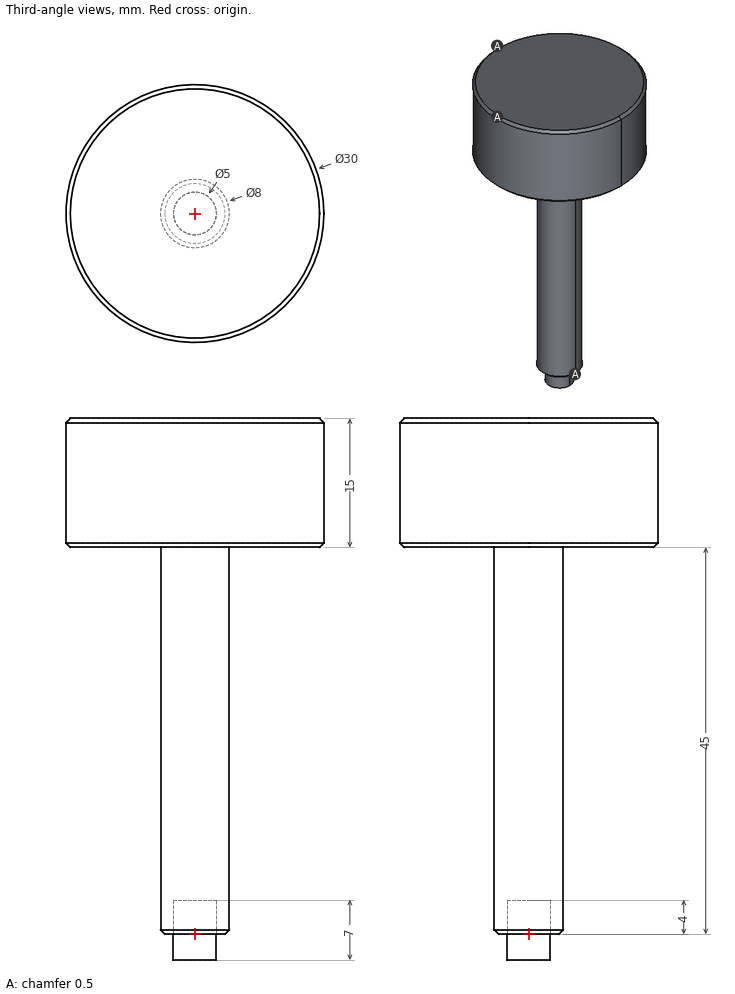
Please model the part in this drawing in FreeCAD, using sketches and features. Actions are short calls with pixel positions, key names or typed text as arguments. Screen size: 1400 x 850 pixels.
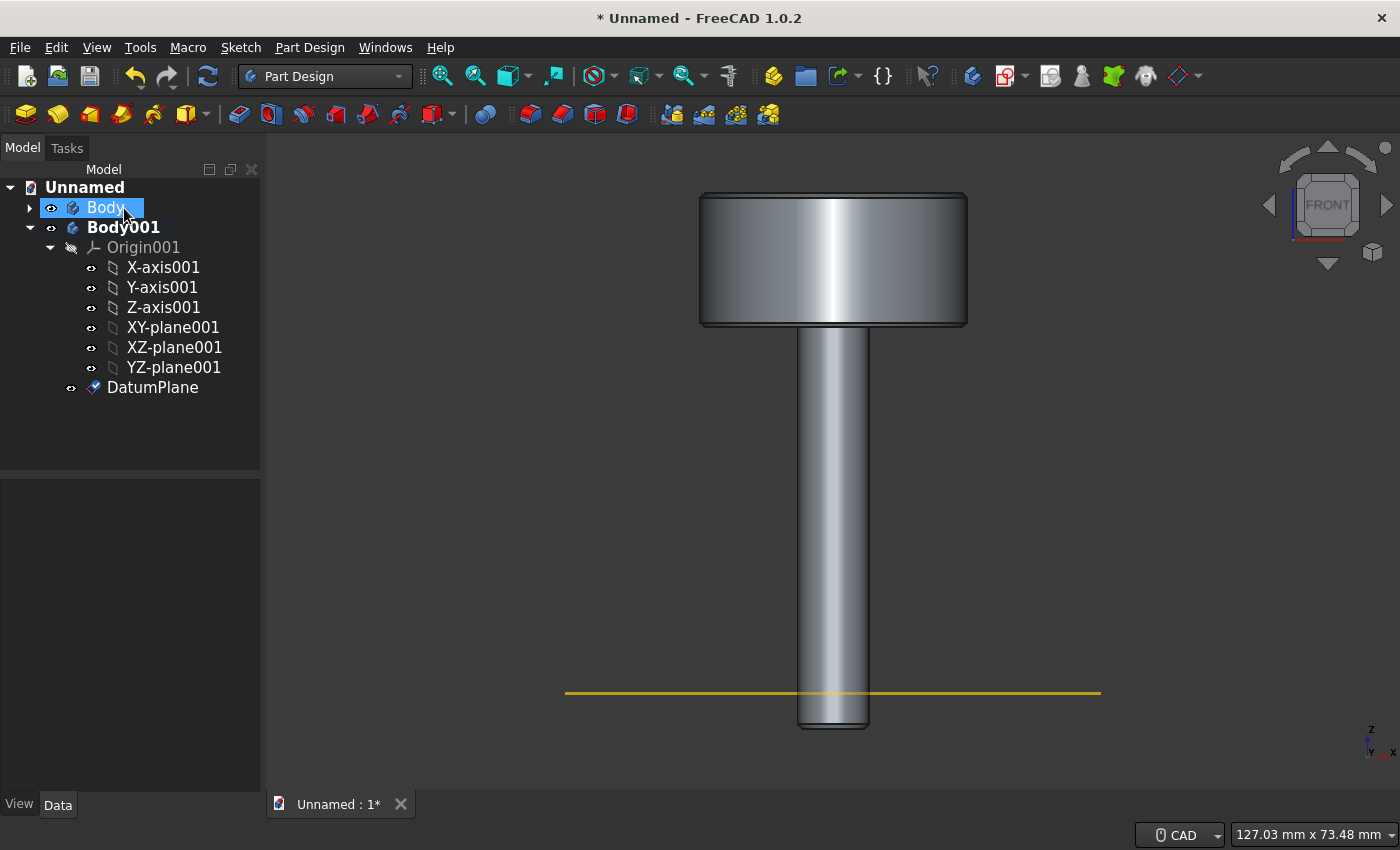
click(116, 388)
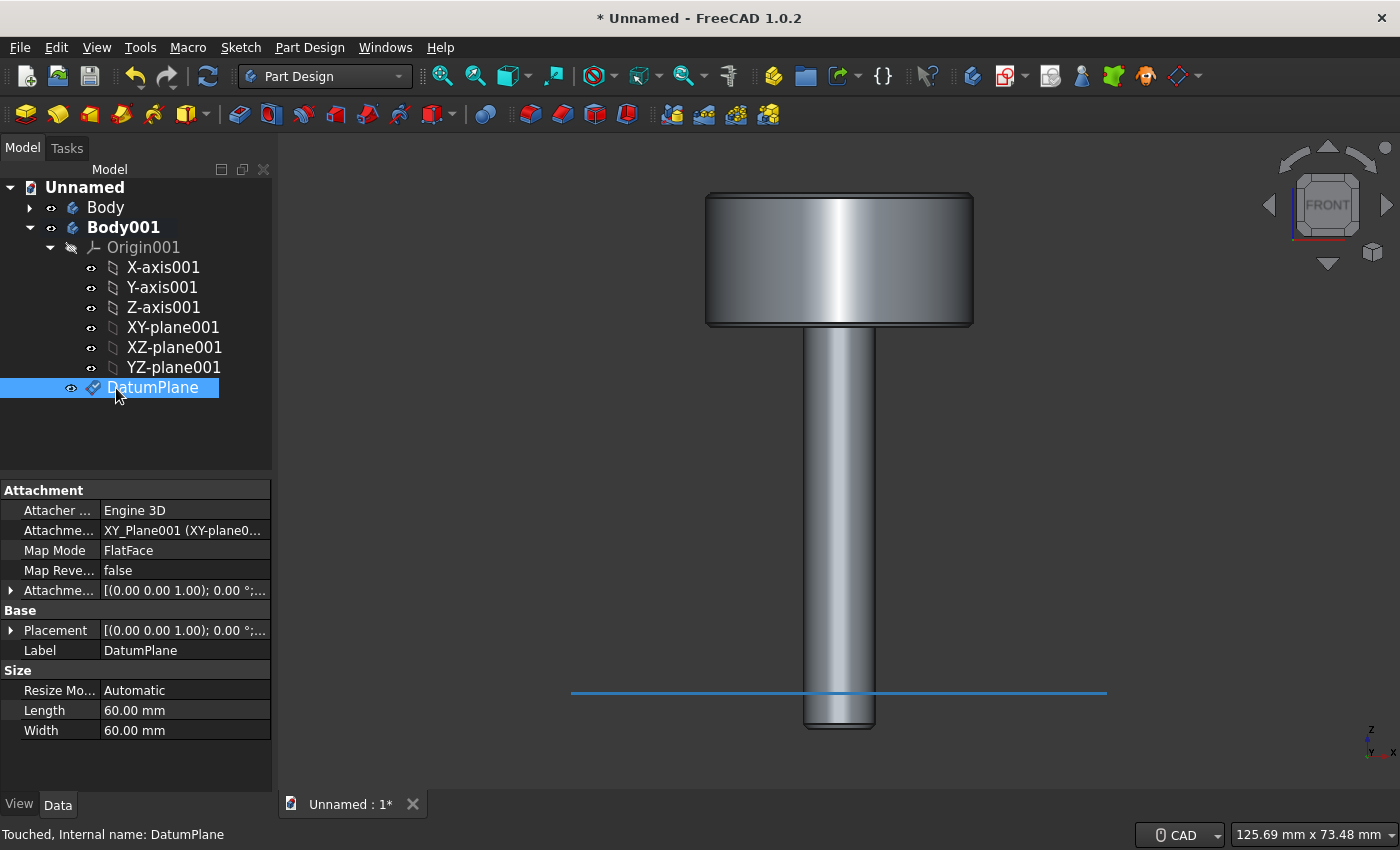
click(1006, 76)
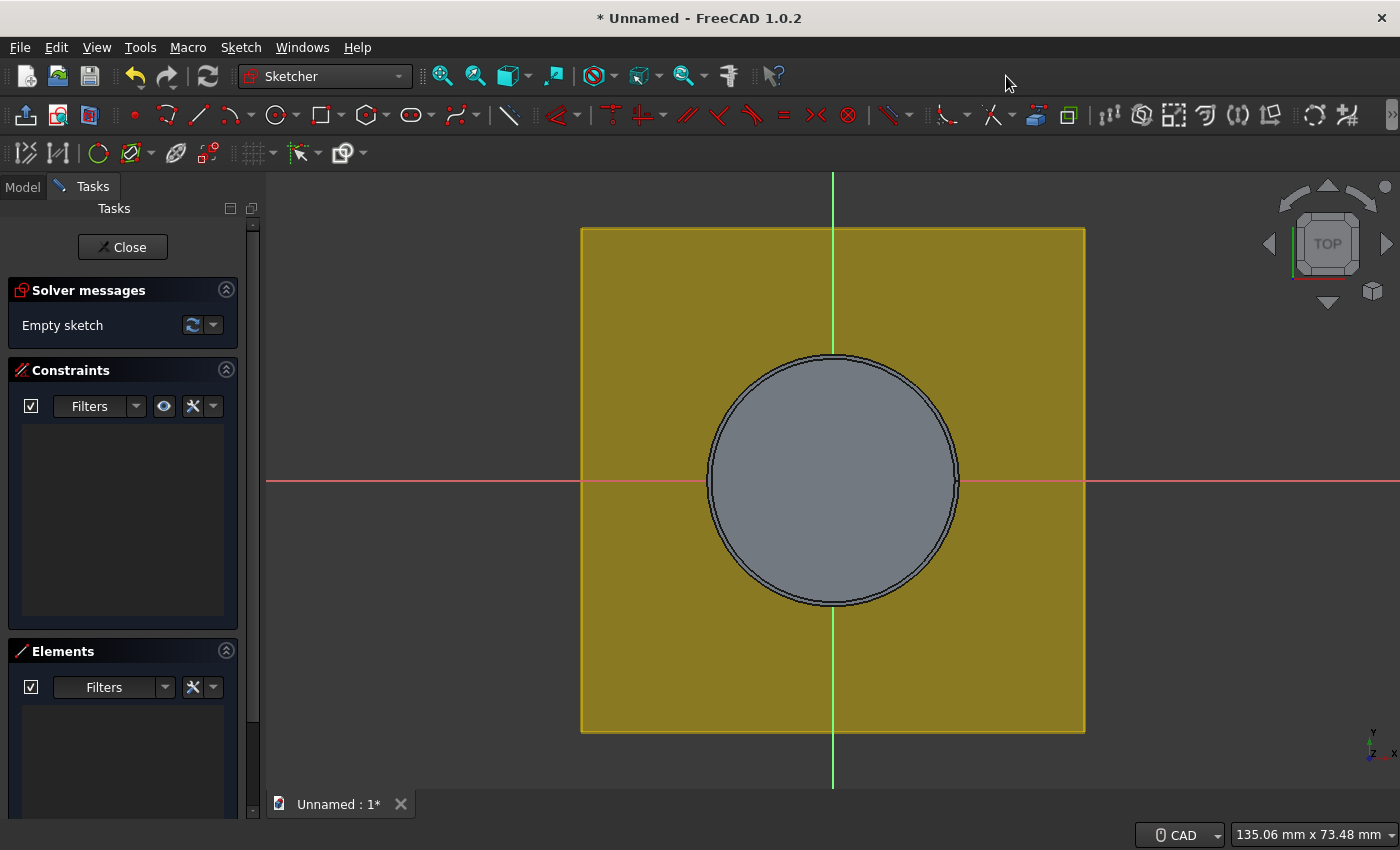
scroll(842, 480, up, 11)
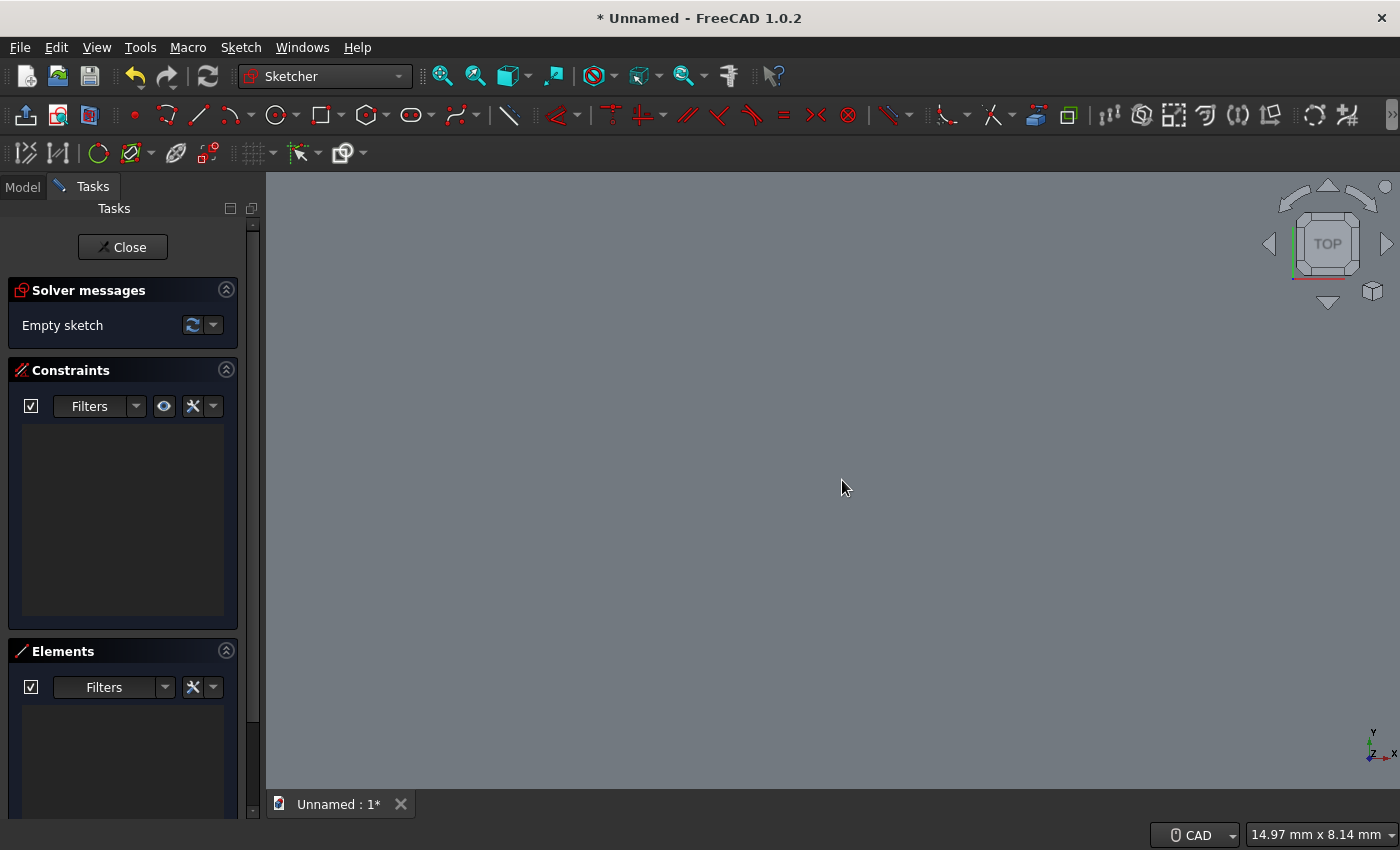
click(276, 116)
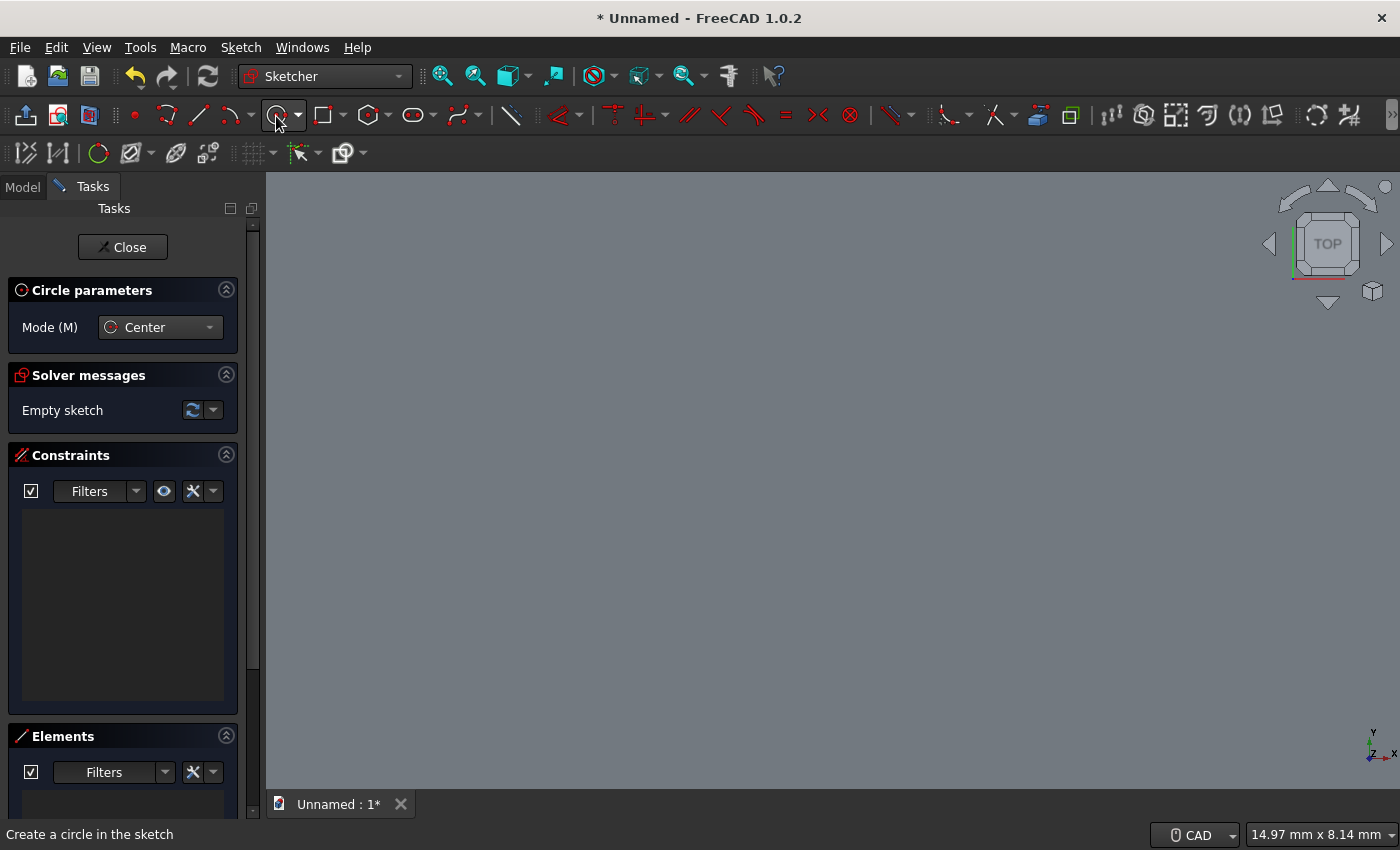
click(757, 480)
move(891, 347)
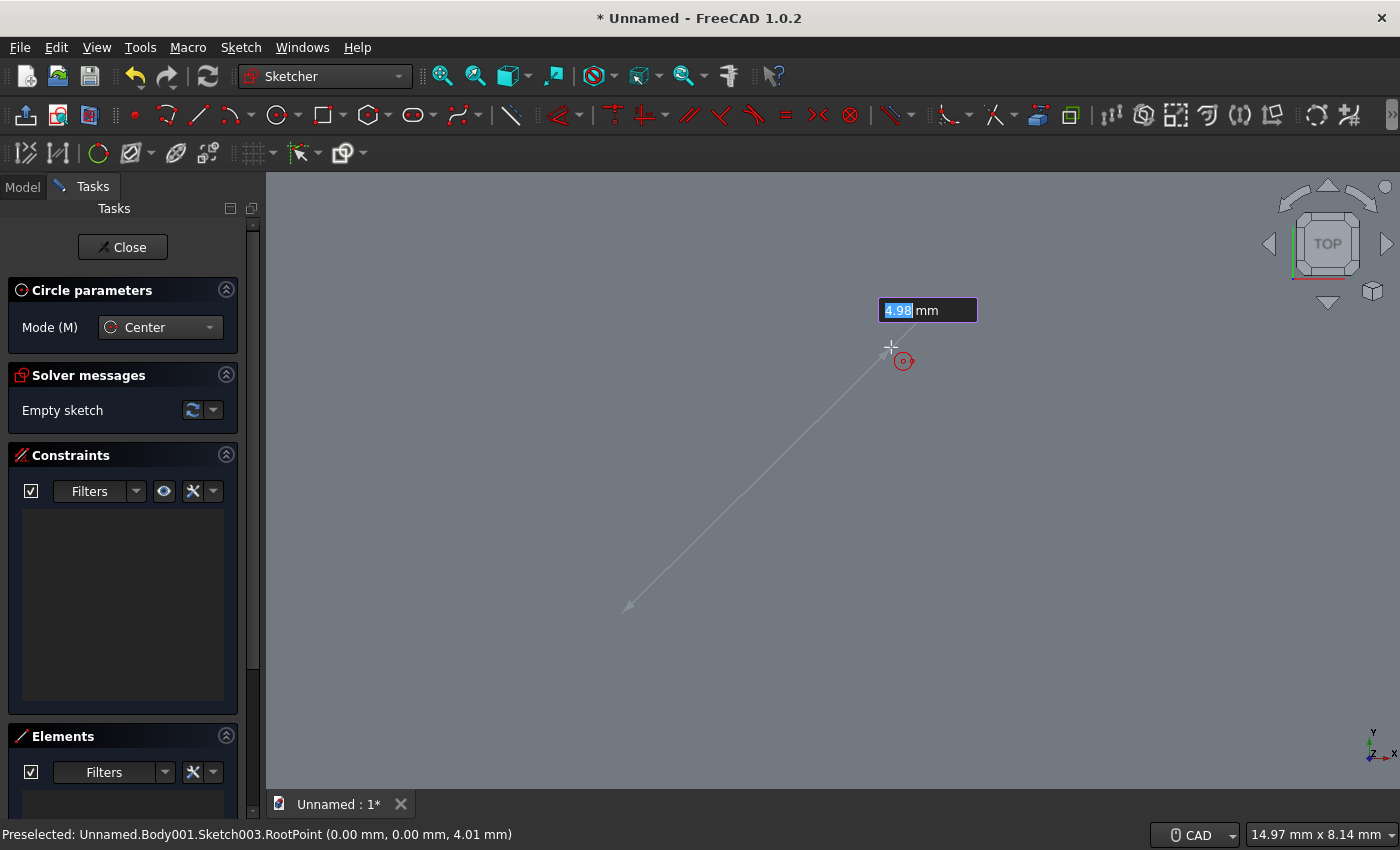
text(5)
key(Return)
key(Escape)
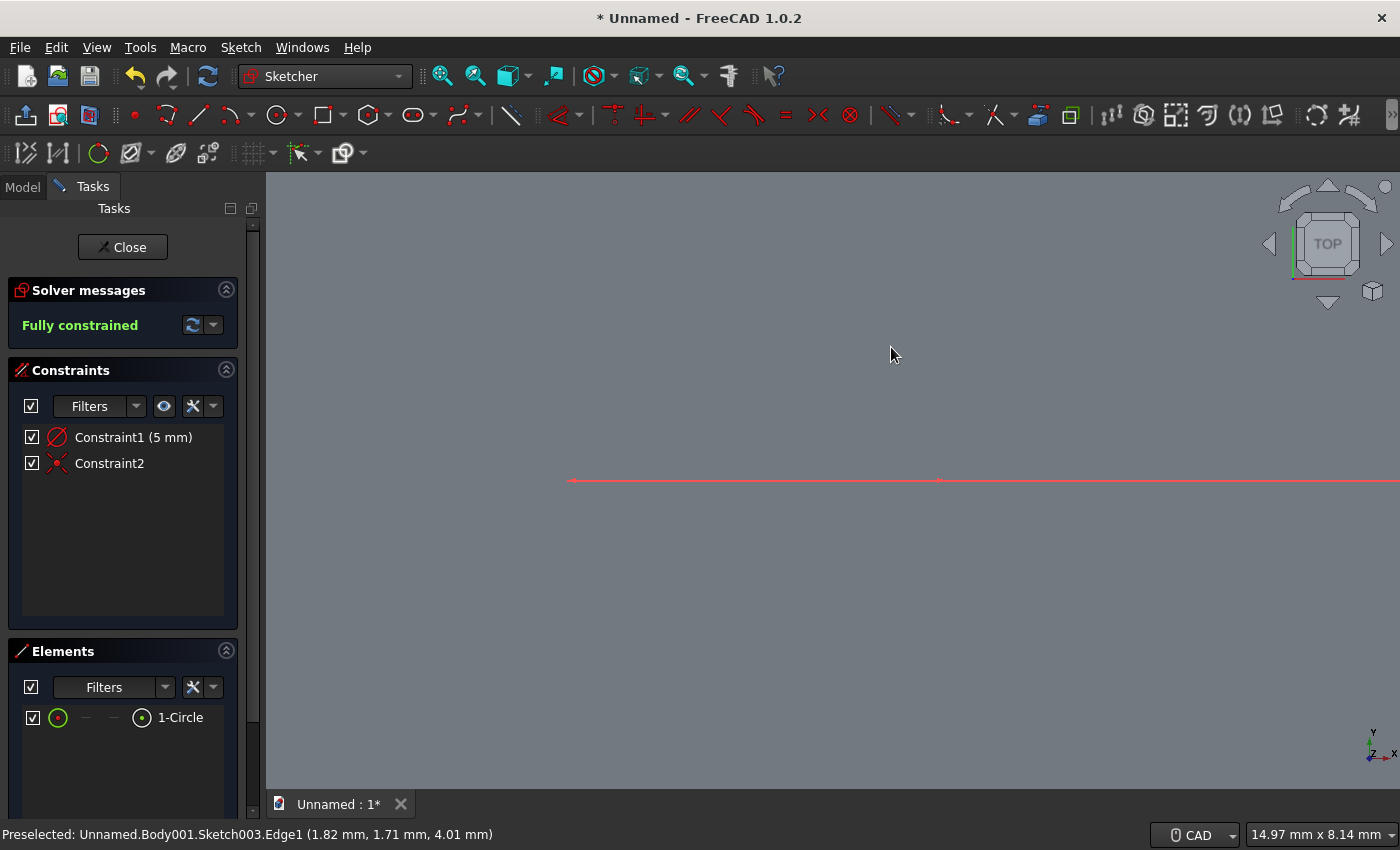
click(123, 247)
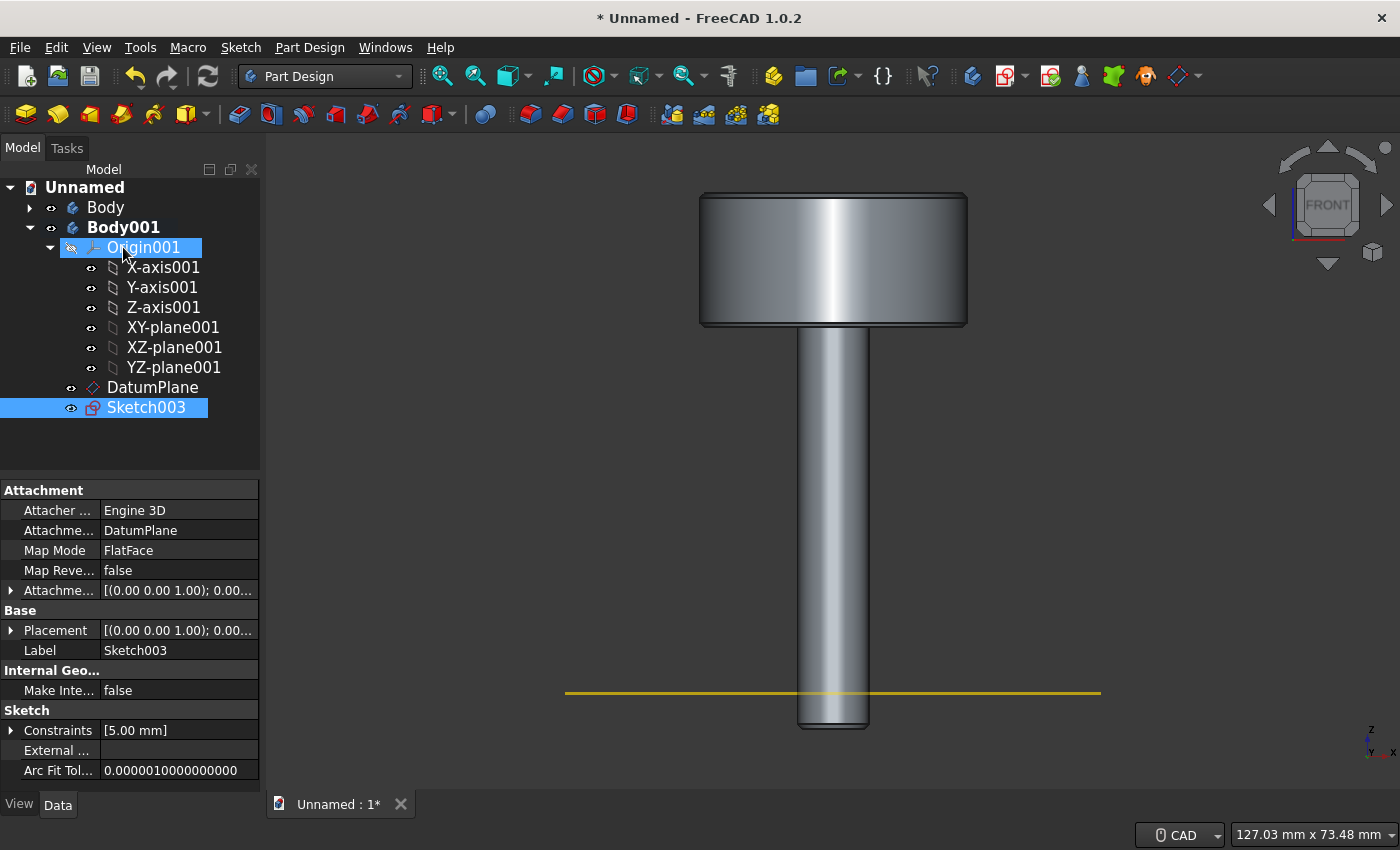
click(26, 114)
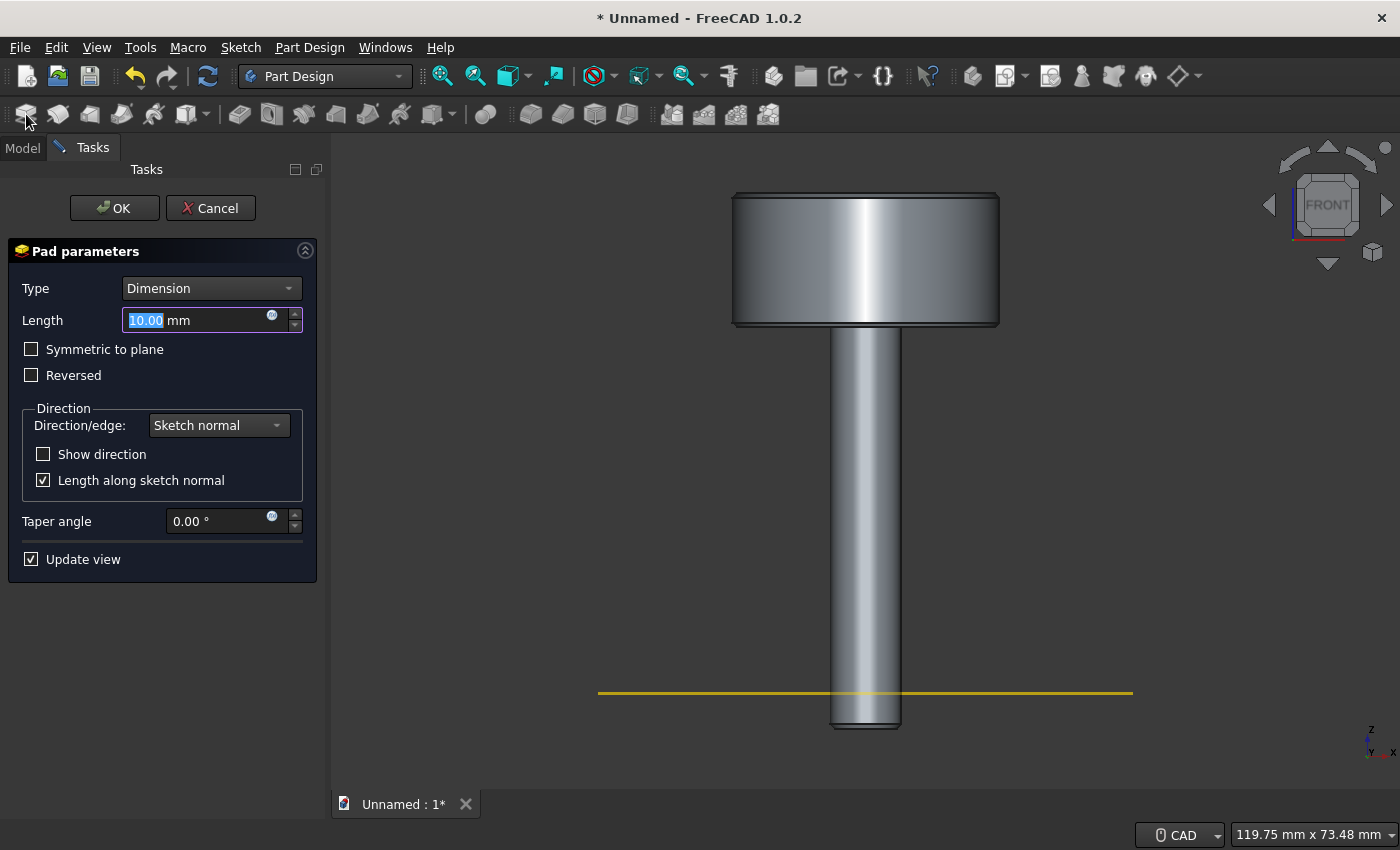
text(7)
key(Tab)